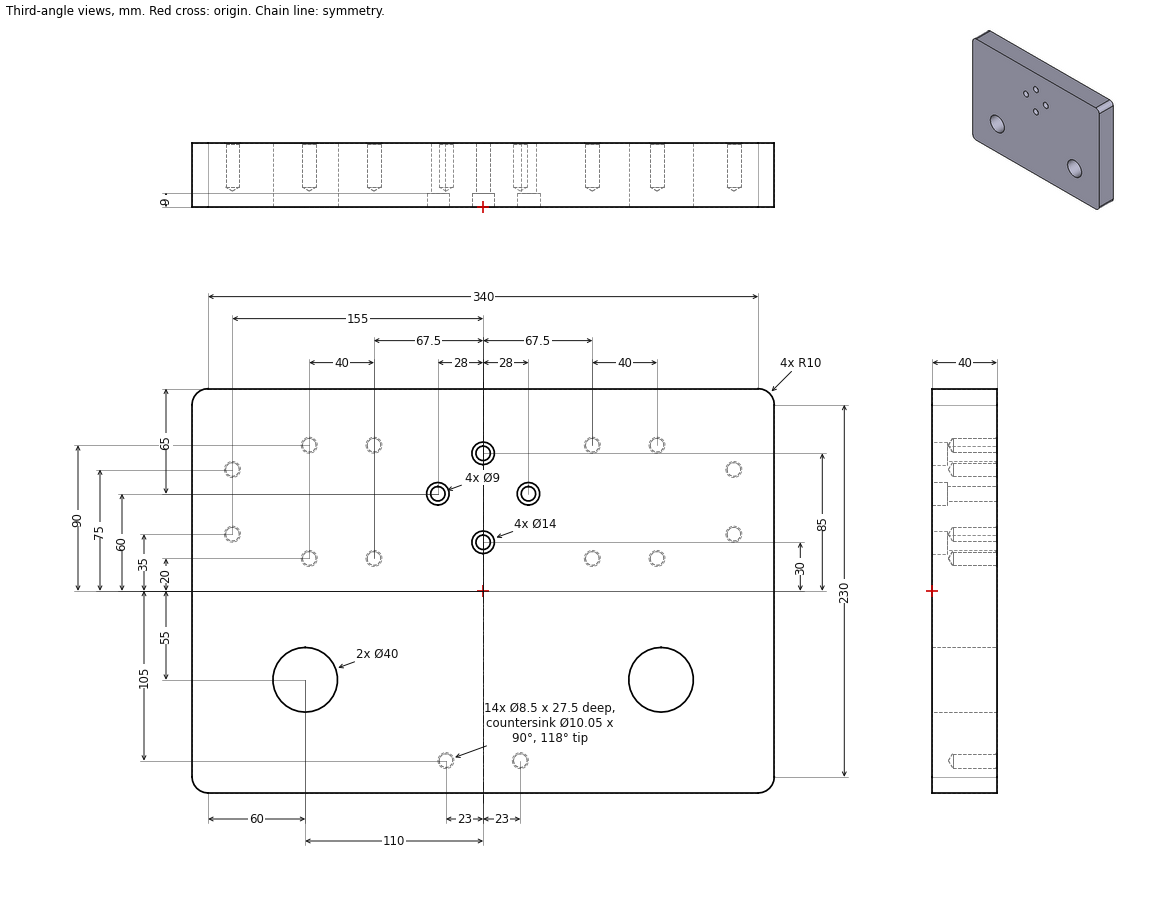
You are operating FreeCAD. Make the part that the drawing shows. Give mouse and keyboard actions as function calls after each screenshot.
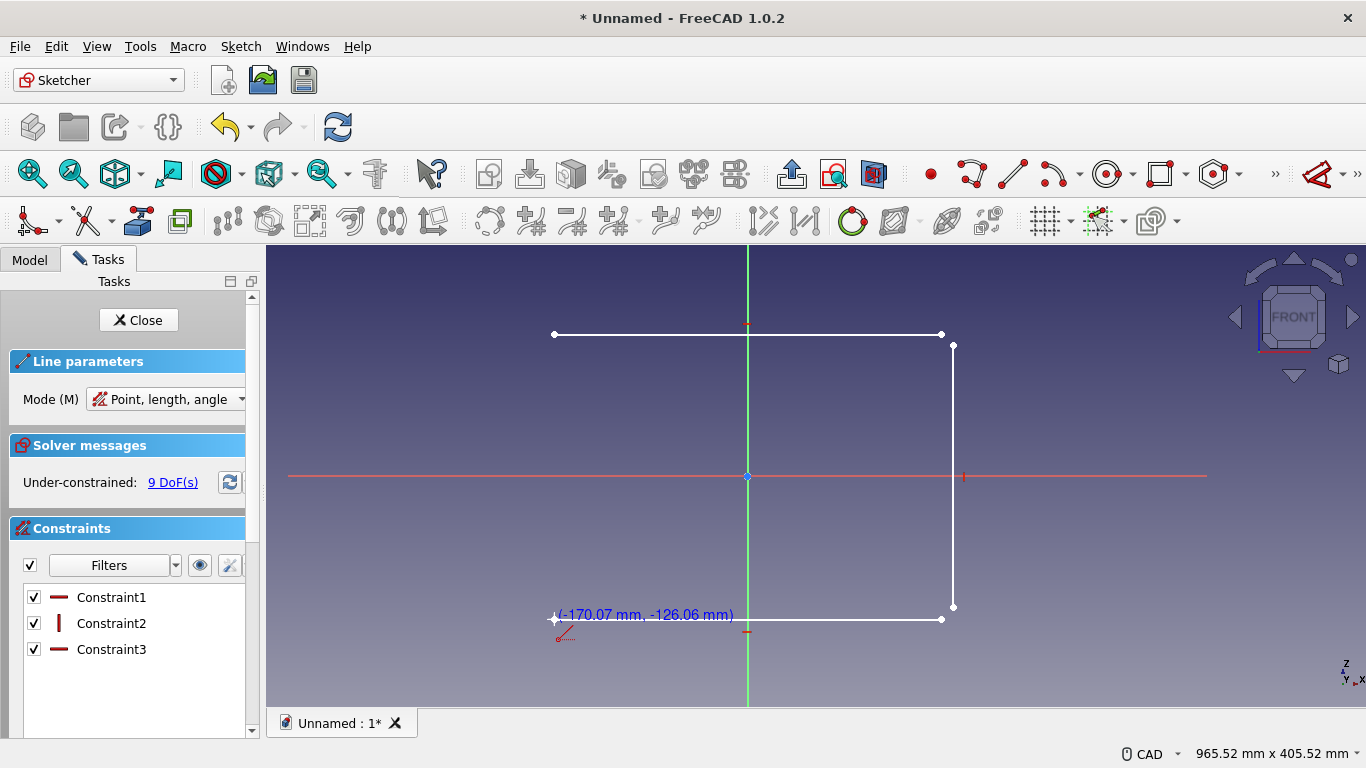
click(543, 607)
click(543, 345)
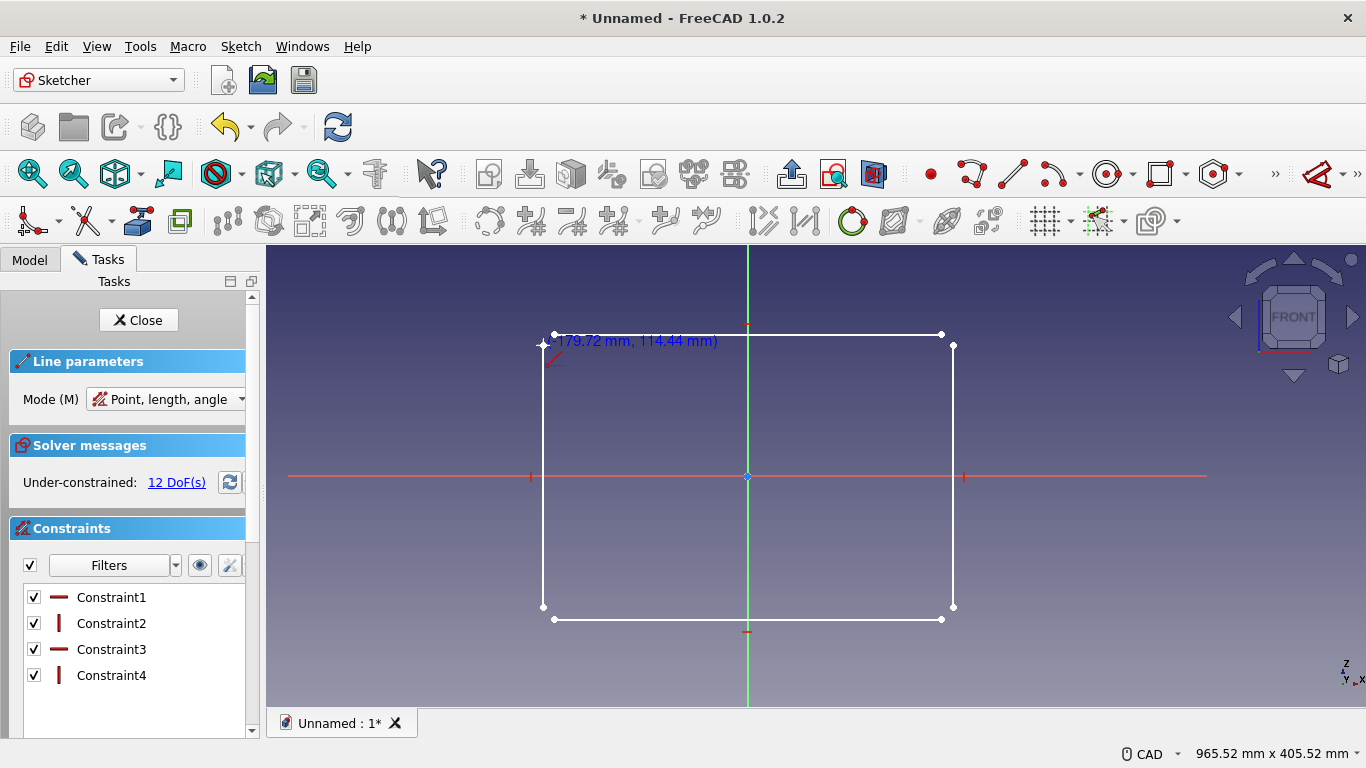
click(1080, 174)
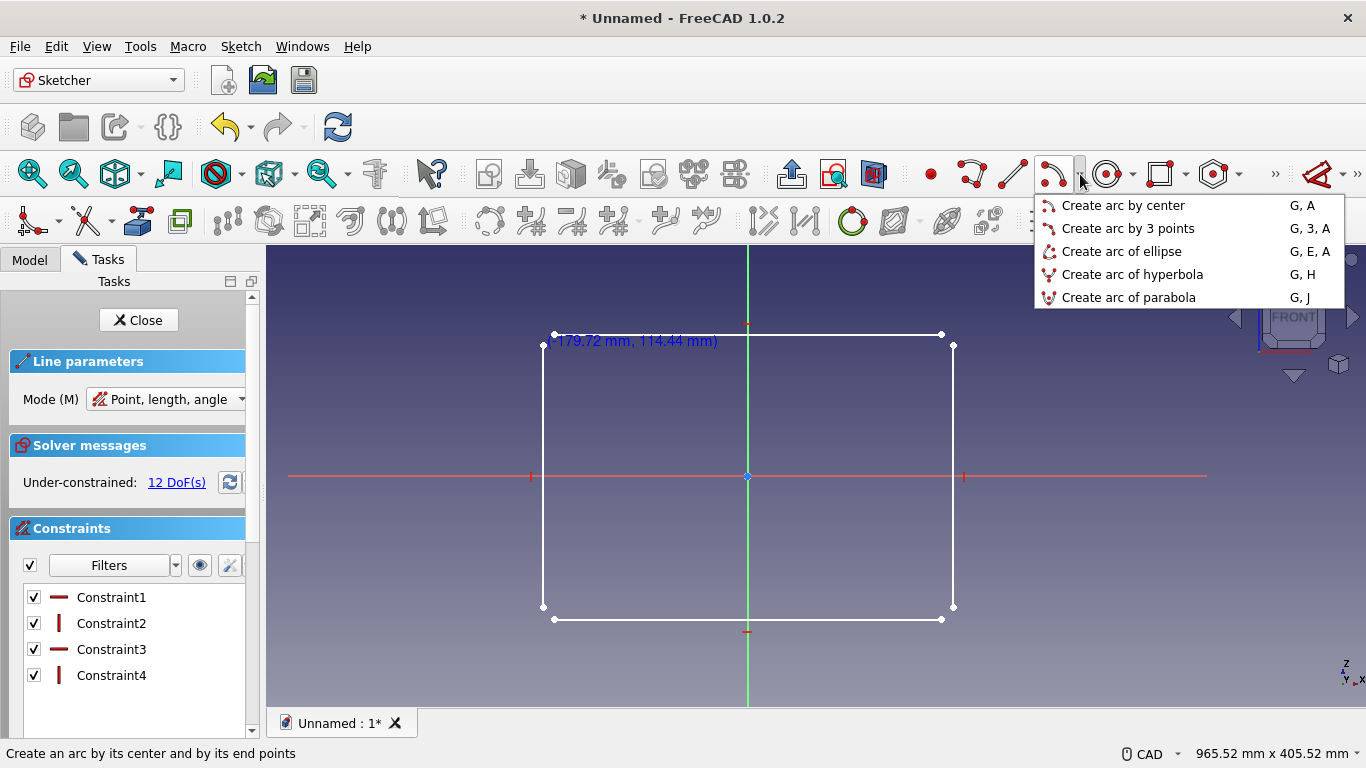
click(1190, 228)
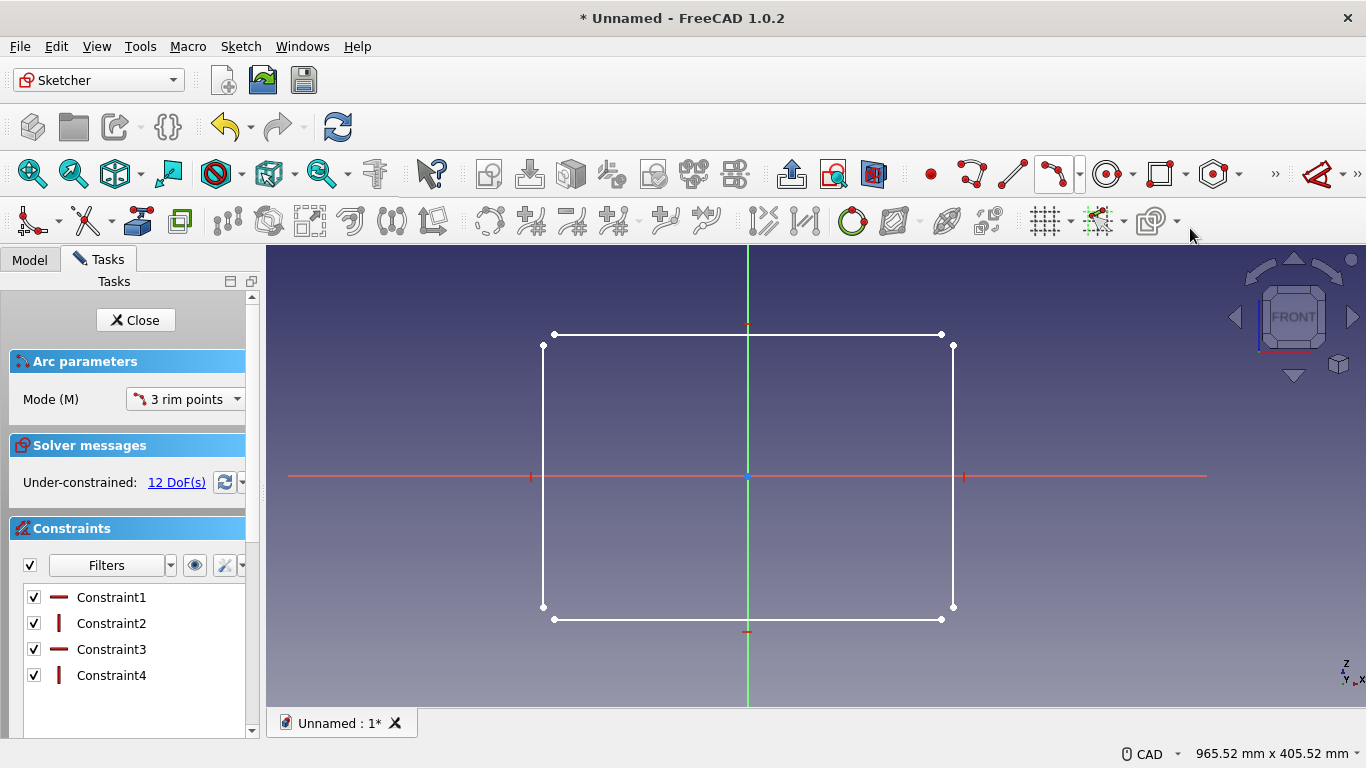
click(941, 335)
click(953, 346)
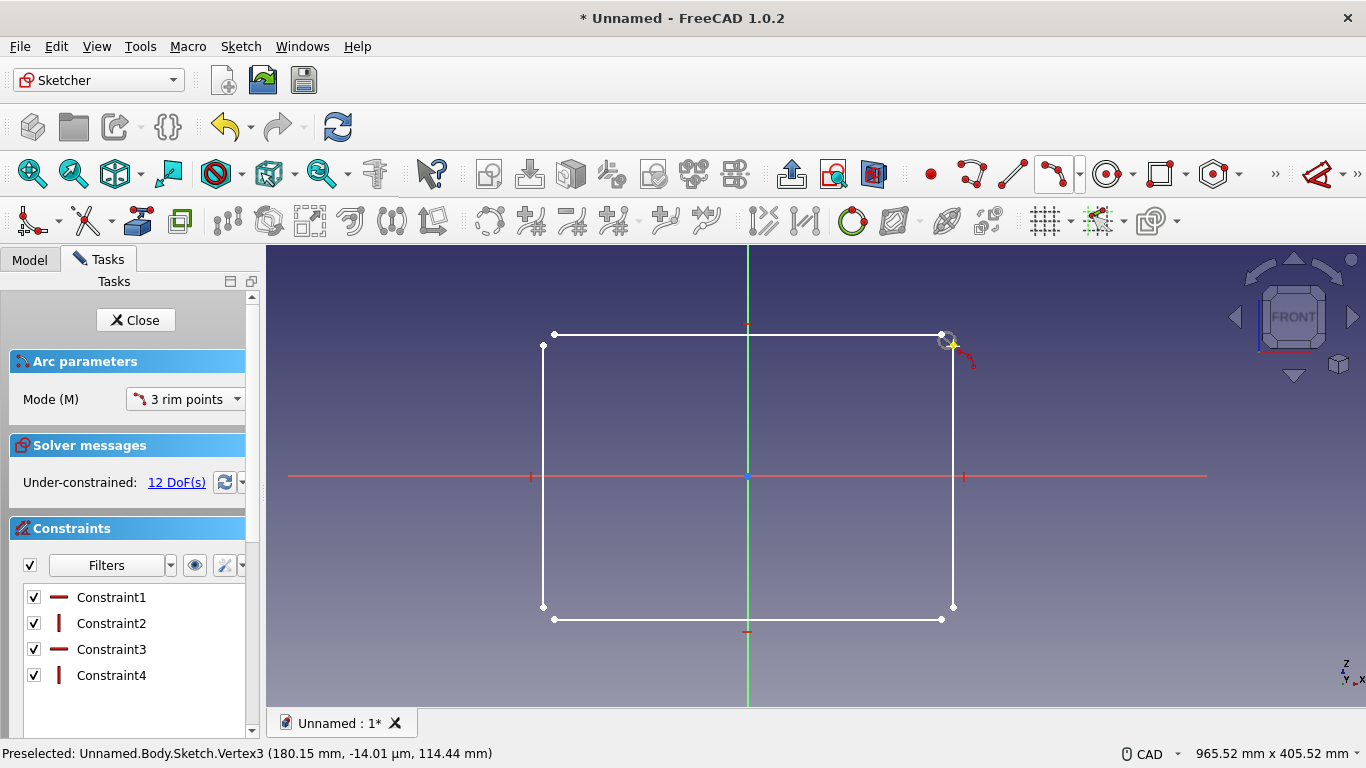
scroll(949, 337, up, 8)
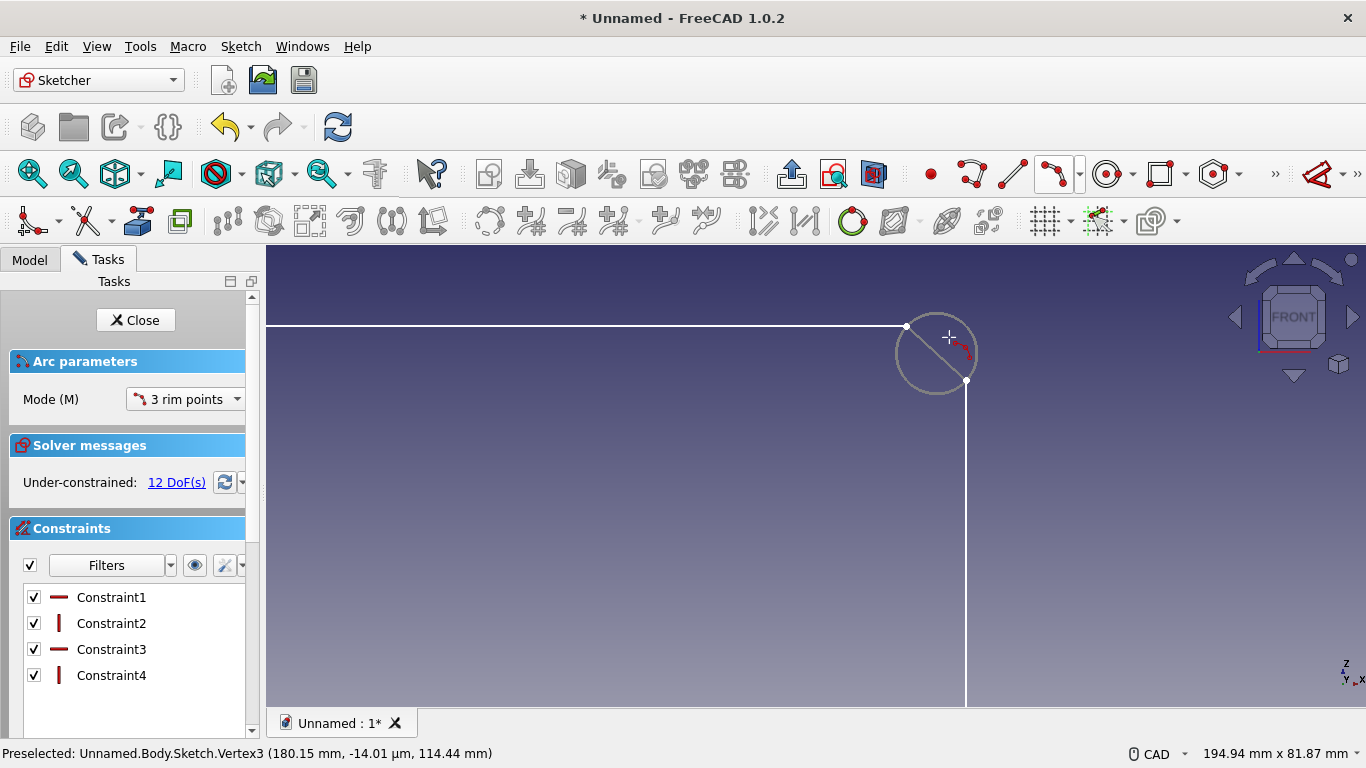
click(949, 338)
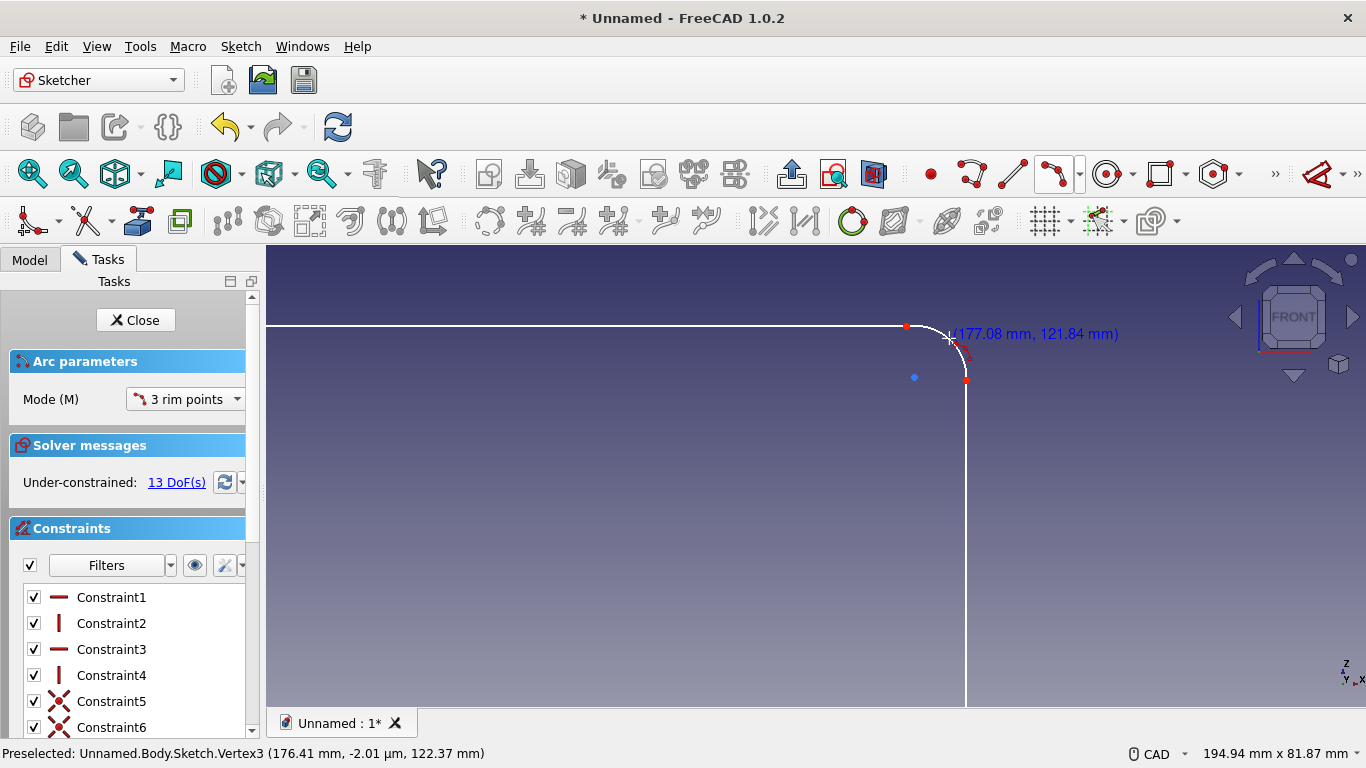
scroll(949, 337, down, 8)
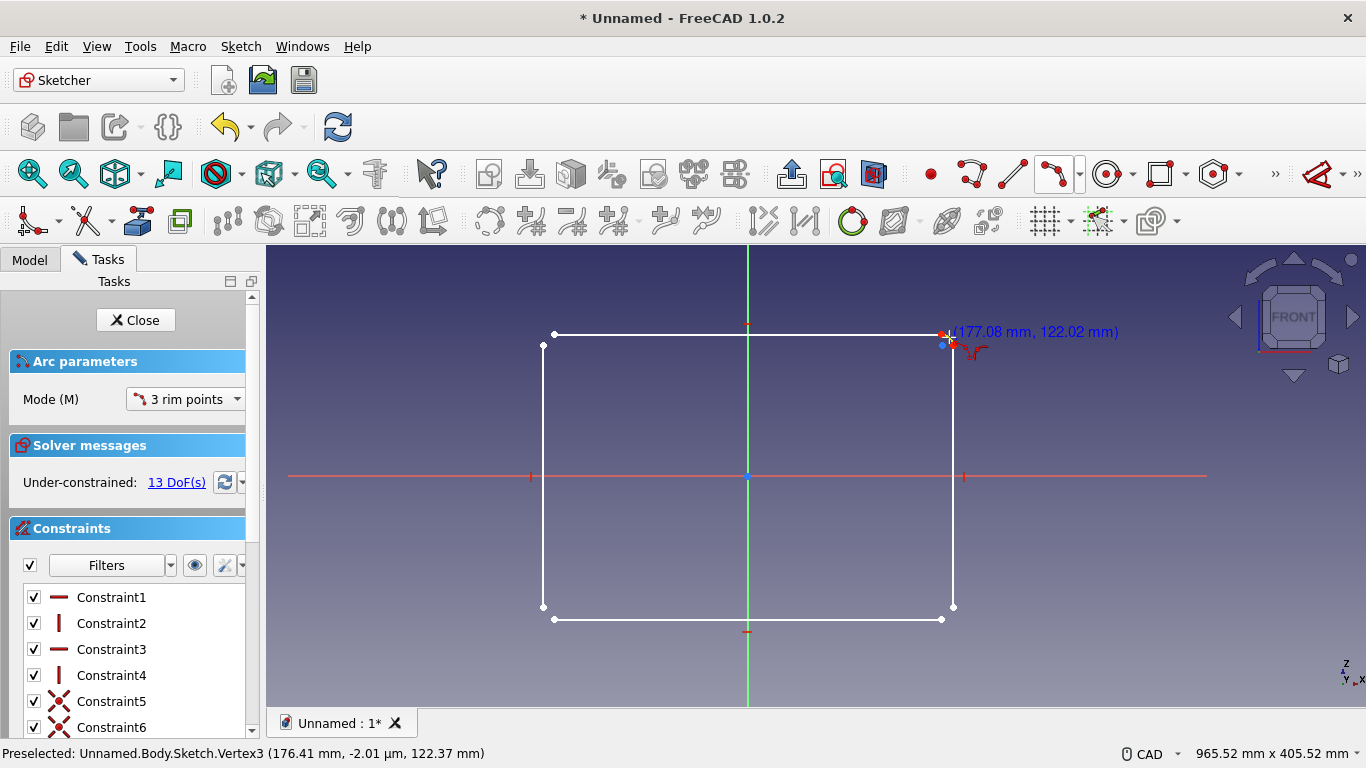
click(953, 608)
click(941, 620)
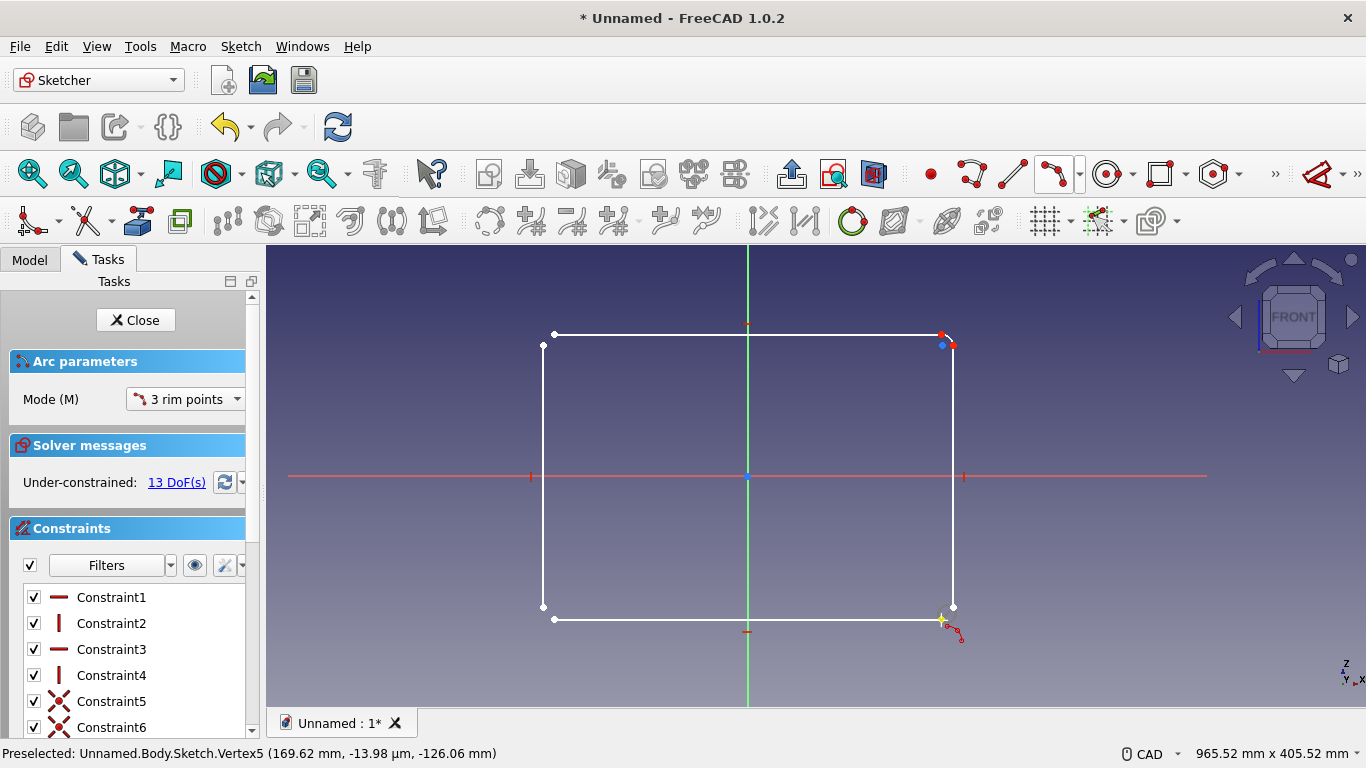
scroll(949, 615, up, 8)